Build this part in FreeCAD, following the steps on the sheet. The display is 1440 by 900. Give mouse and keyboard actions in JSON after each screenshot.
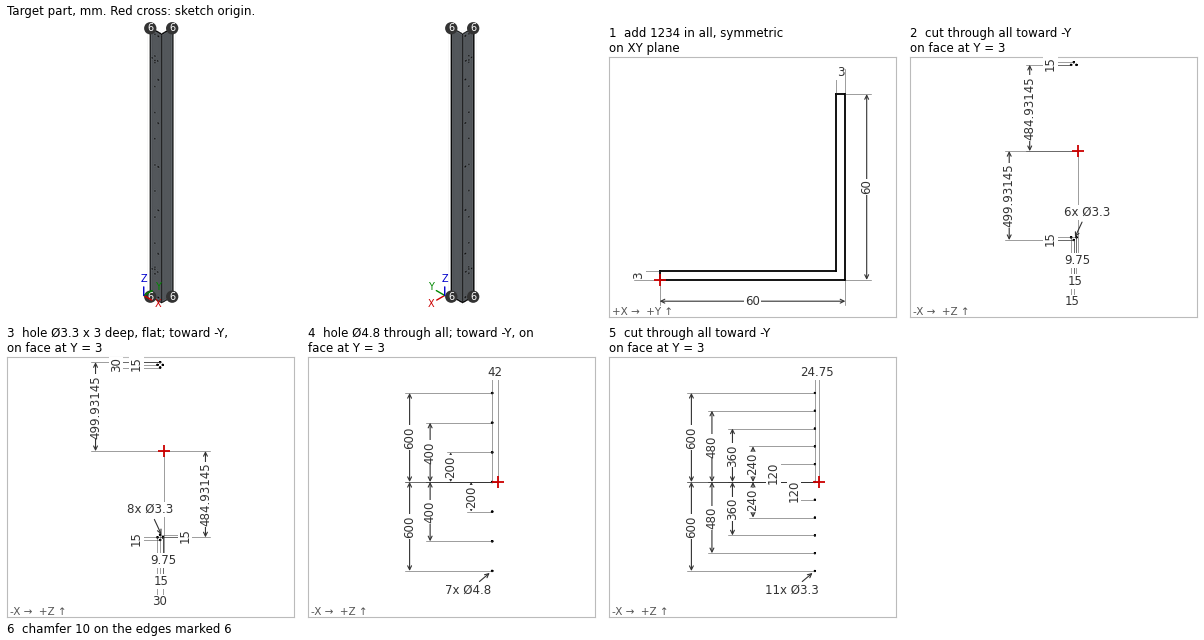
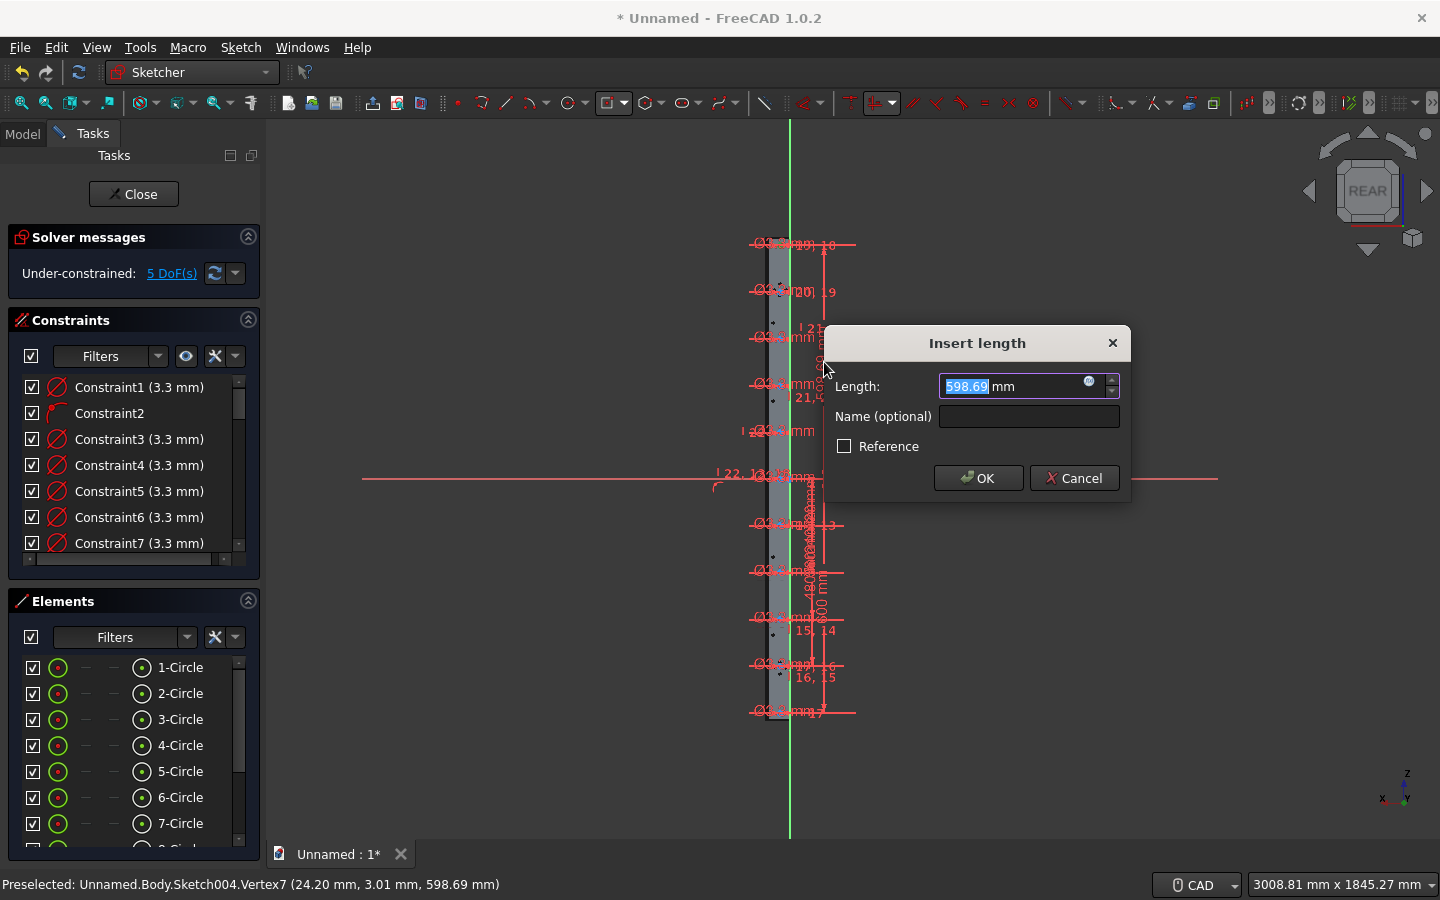
{"action": "type", "text": "600"}
{"action": "key", "text": "Return"}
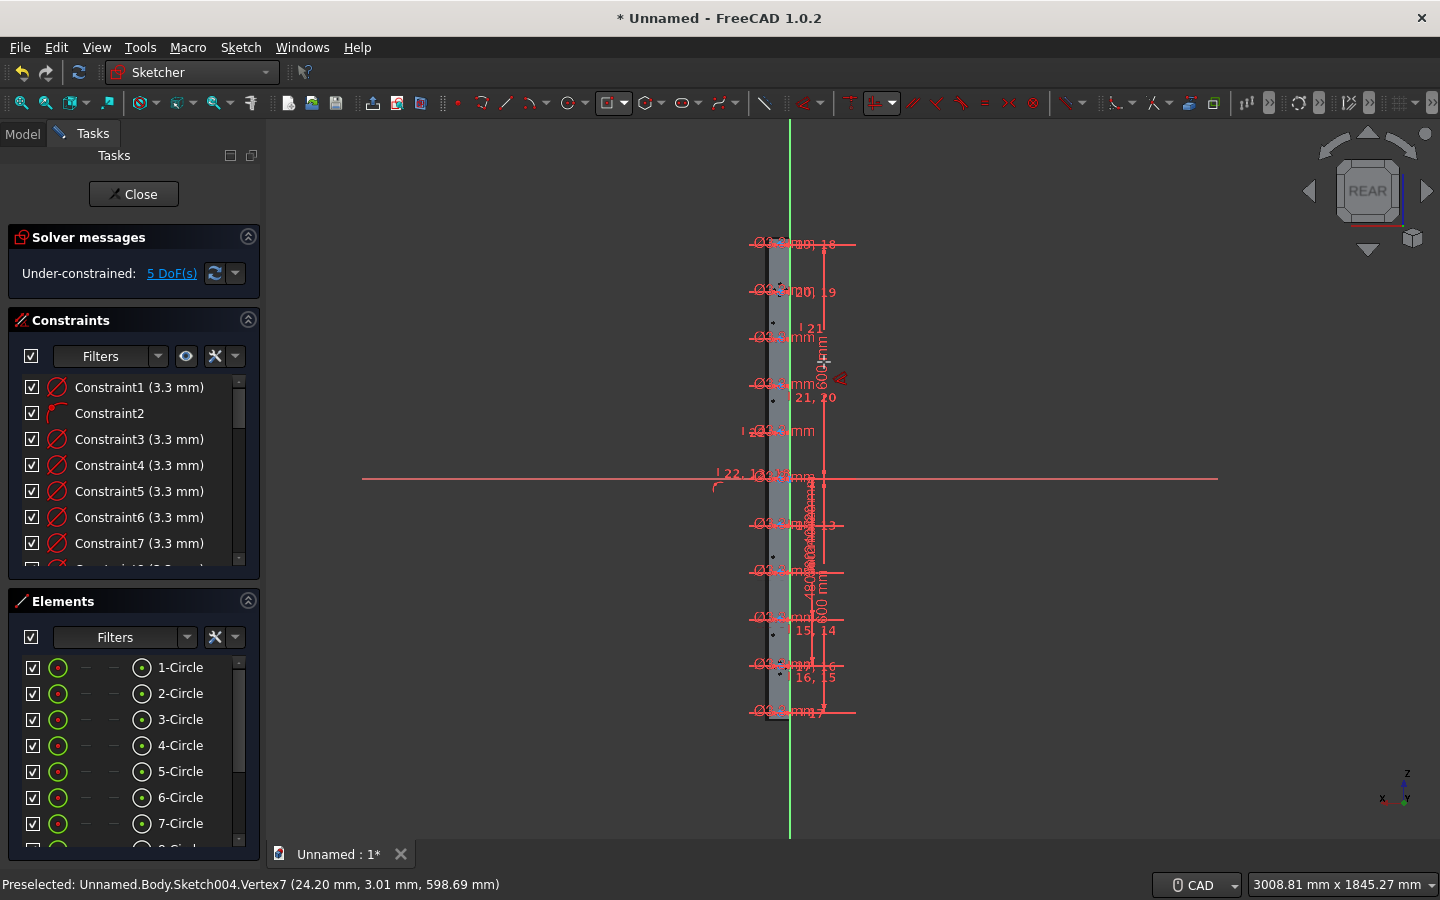
{"action": "left_click", "coordinate": [780, 292]}
{"action": "left_click", "coordinate": [824, 386]}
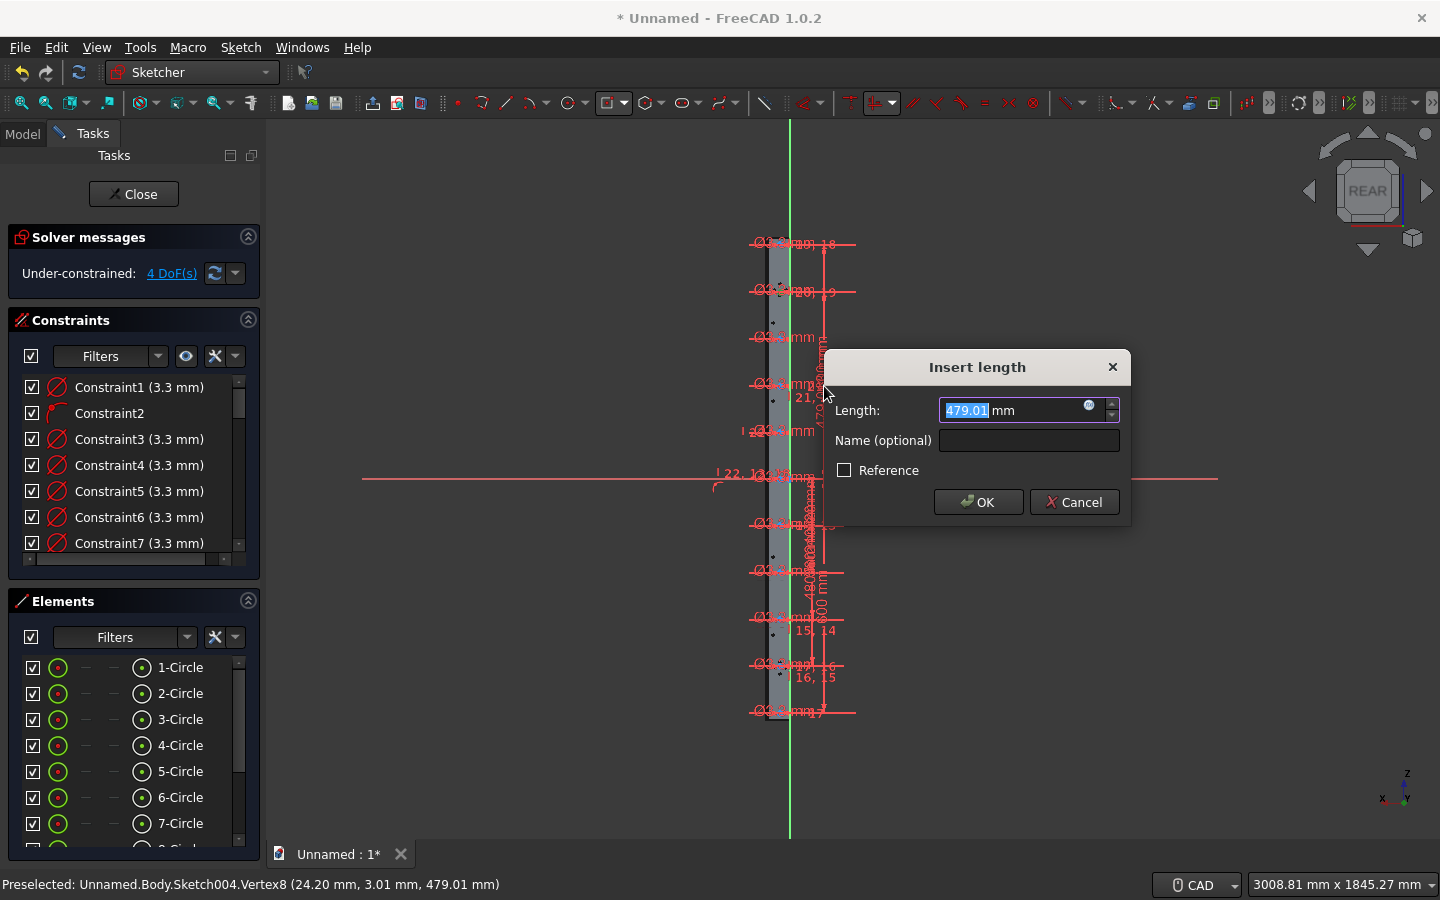
{"action": "type", "text": "480"}
{"action": "key", "text": "Return"}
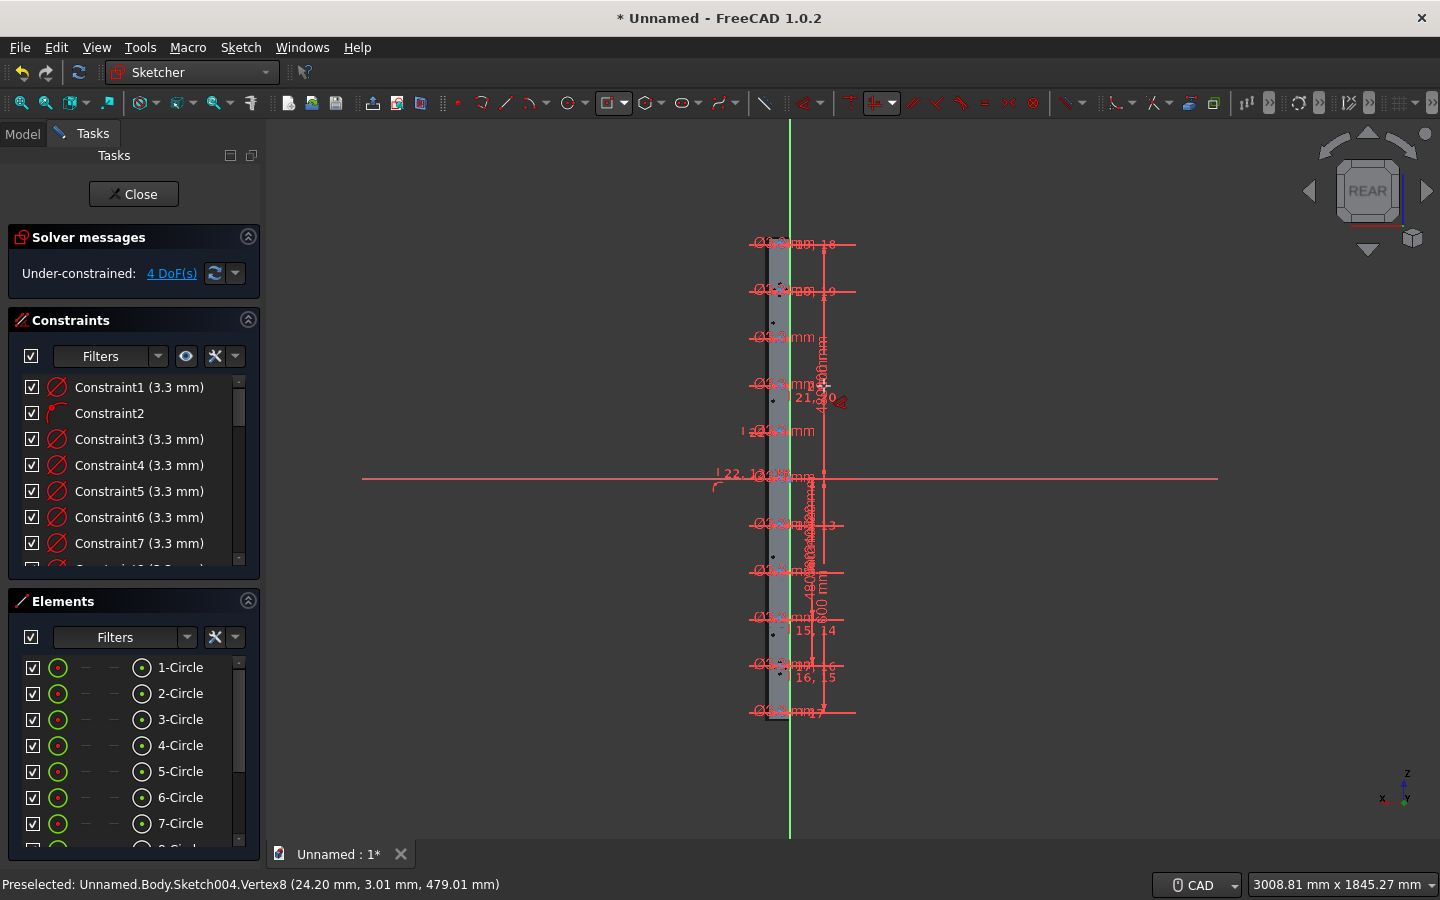
{"action": "left_click", "coordinate": [780, 339]}
{"action": "left_click", "coordinate": [824, 409]}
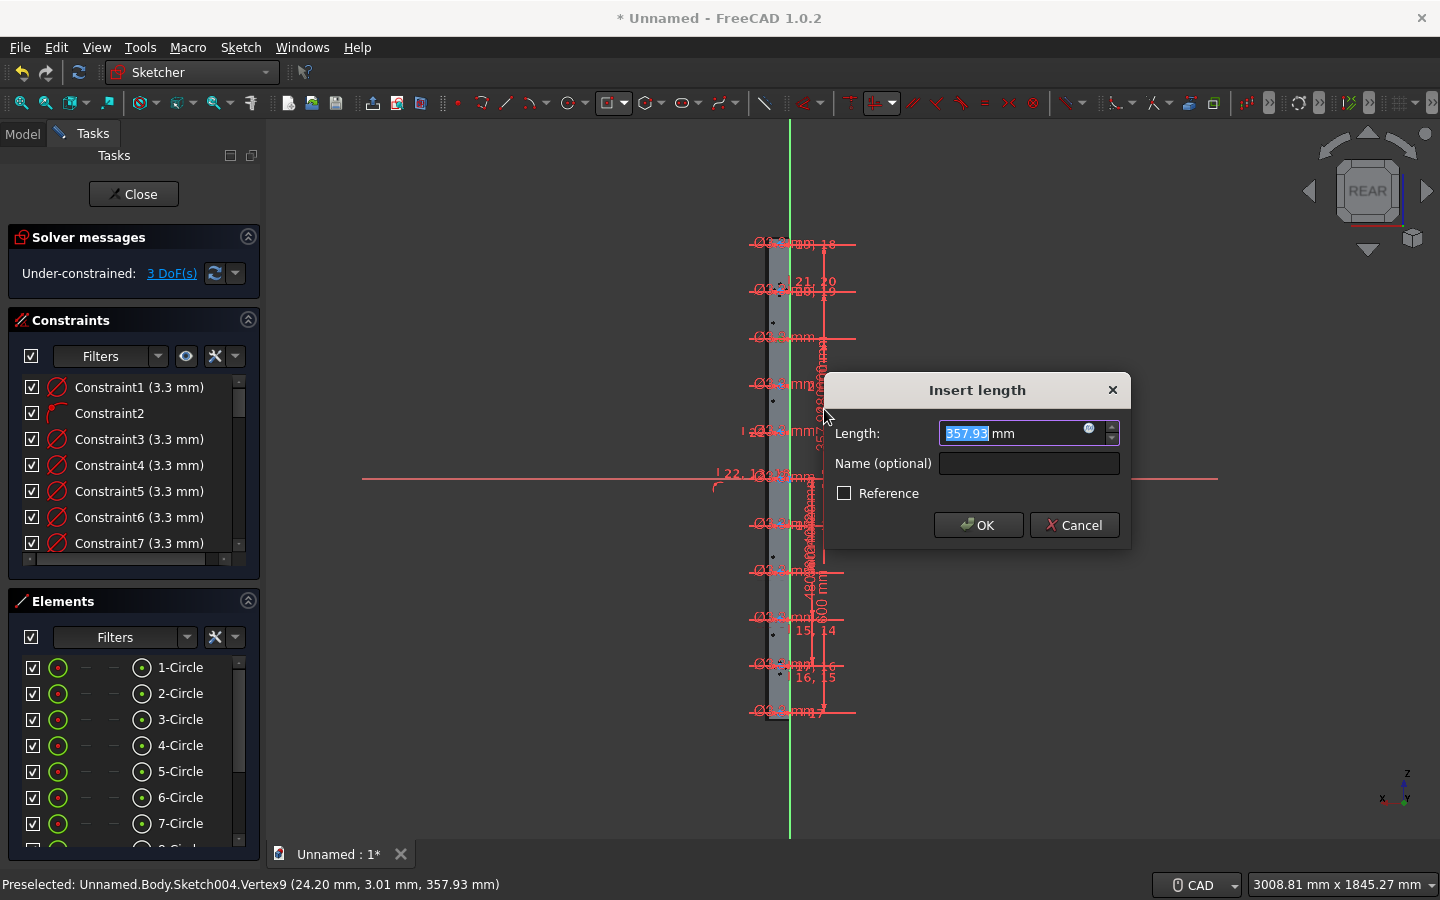
{"action": "type", "text": "360"}
{"action": "key", "text": "Return"}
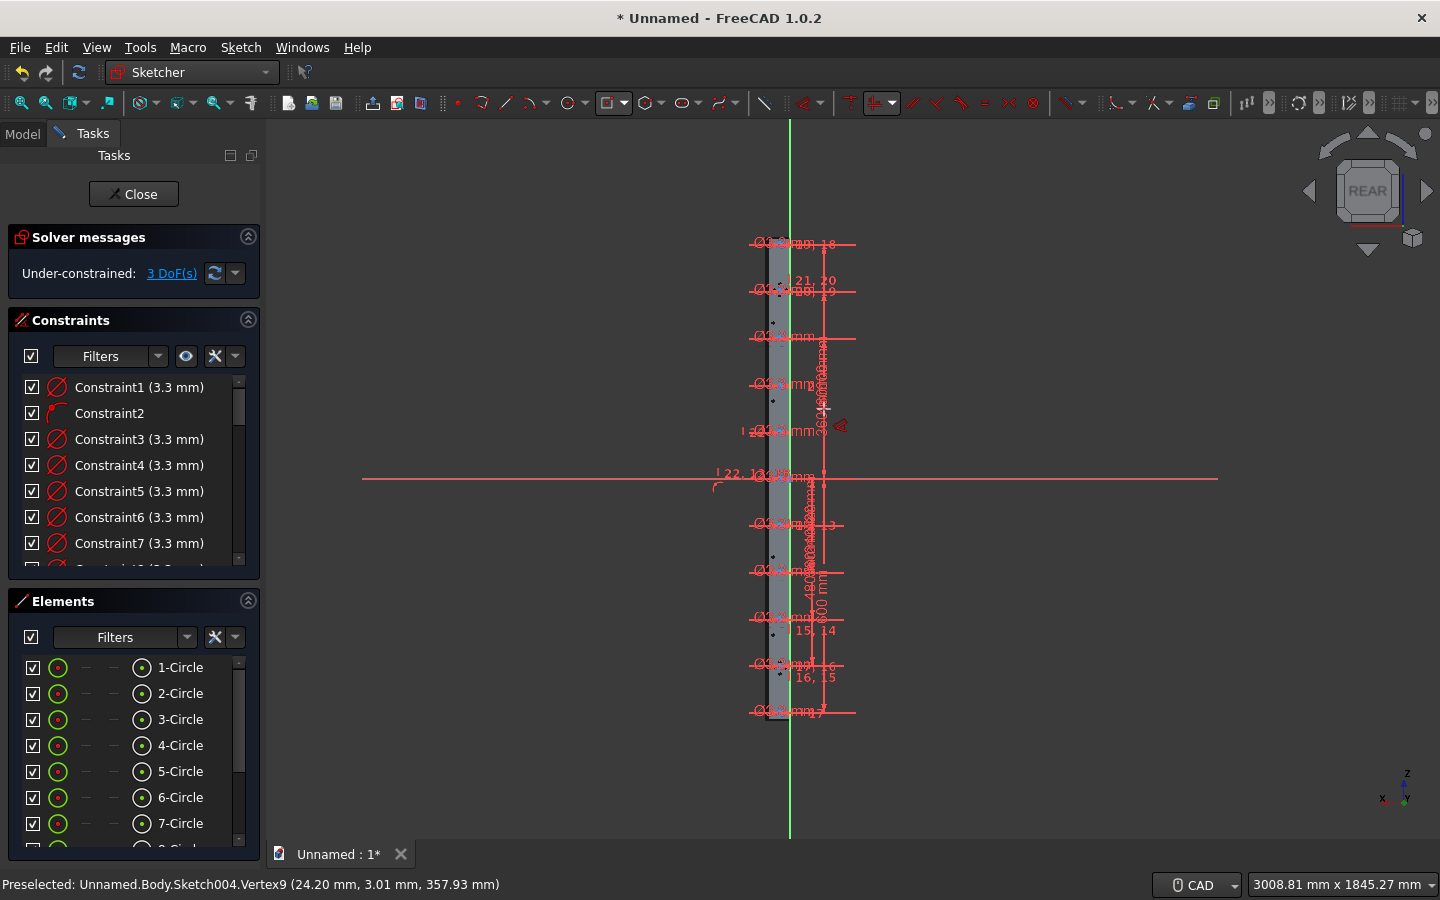
{"action": "left_click", "coordinate": [780, 386]}
{"action": "left_click", "coordinate": [824, 433]}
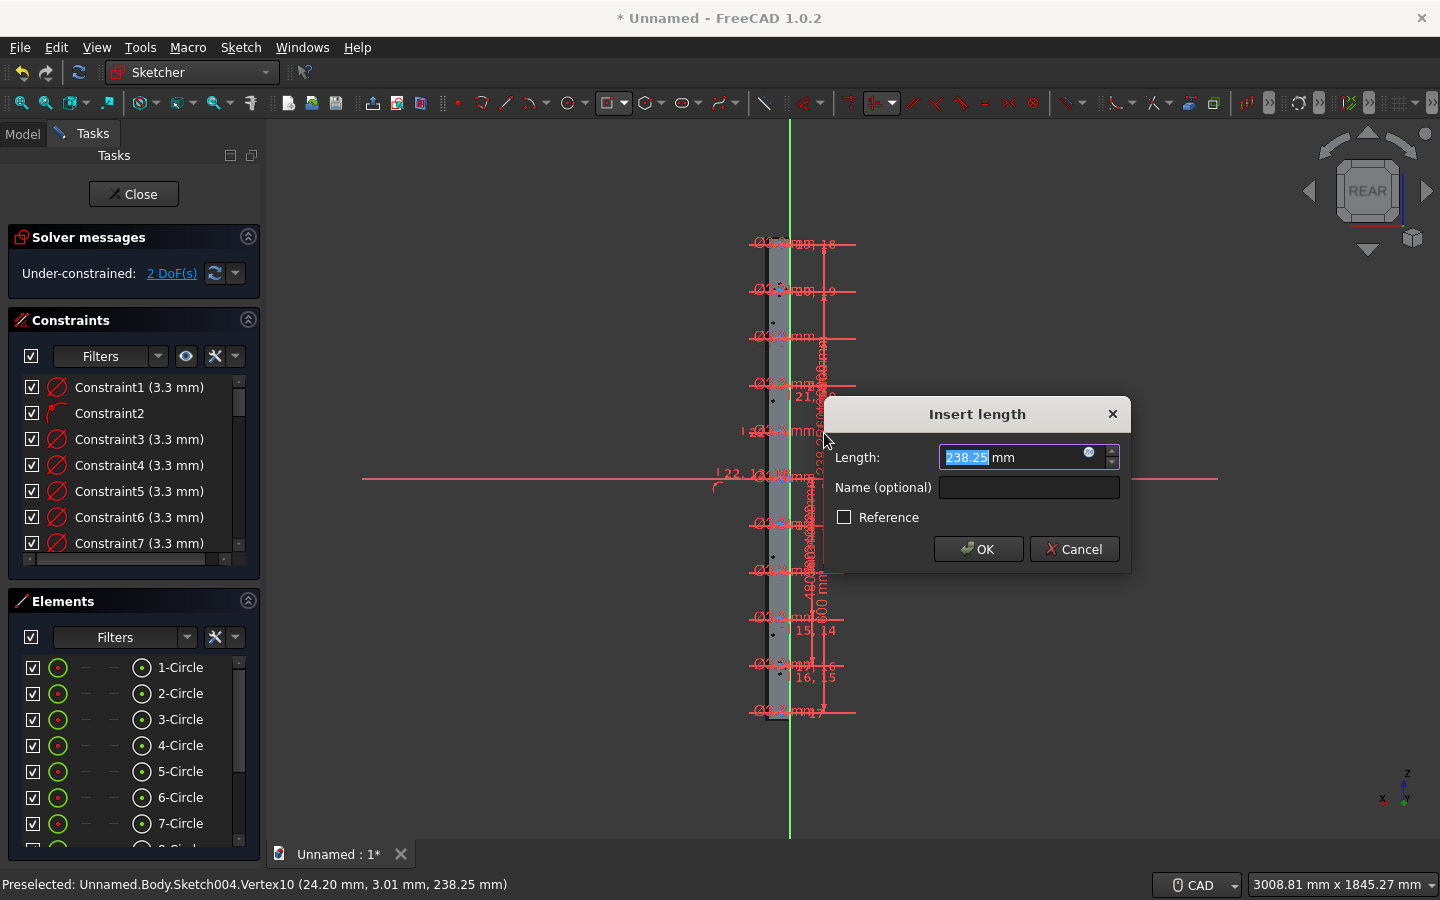
{"action": "type", "text": "240"}
{"action": "key", "text": "Return"}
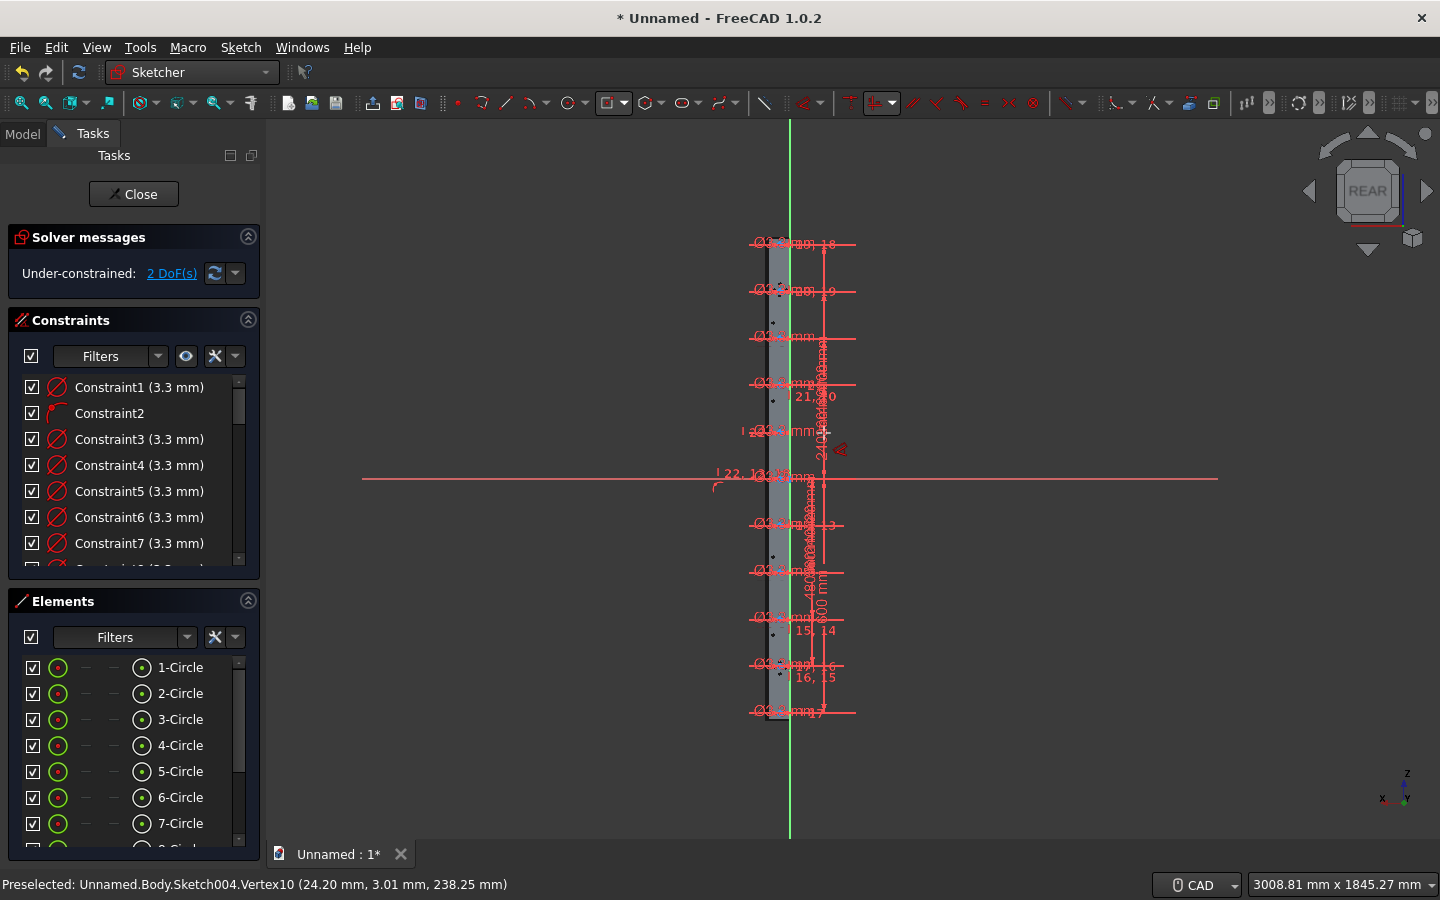
{"action": "left_click", "coordinate": [780, 433]}
{"action": "left_click", "coordinate": [824, 456]}